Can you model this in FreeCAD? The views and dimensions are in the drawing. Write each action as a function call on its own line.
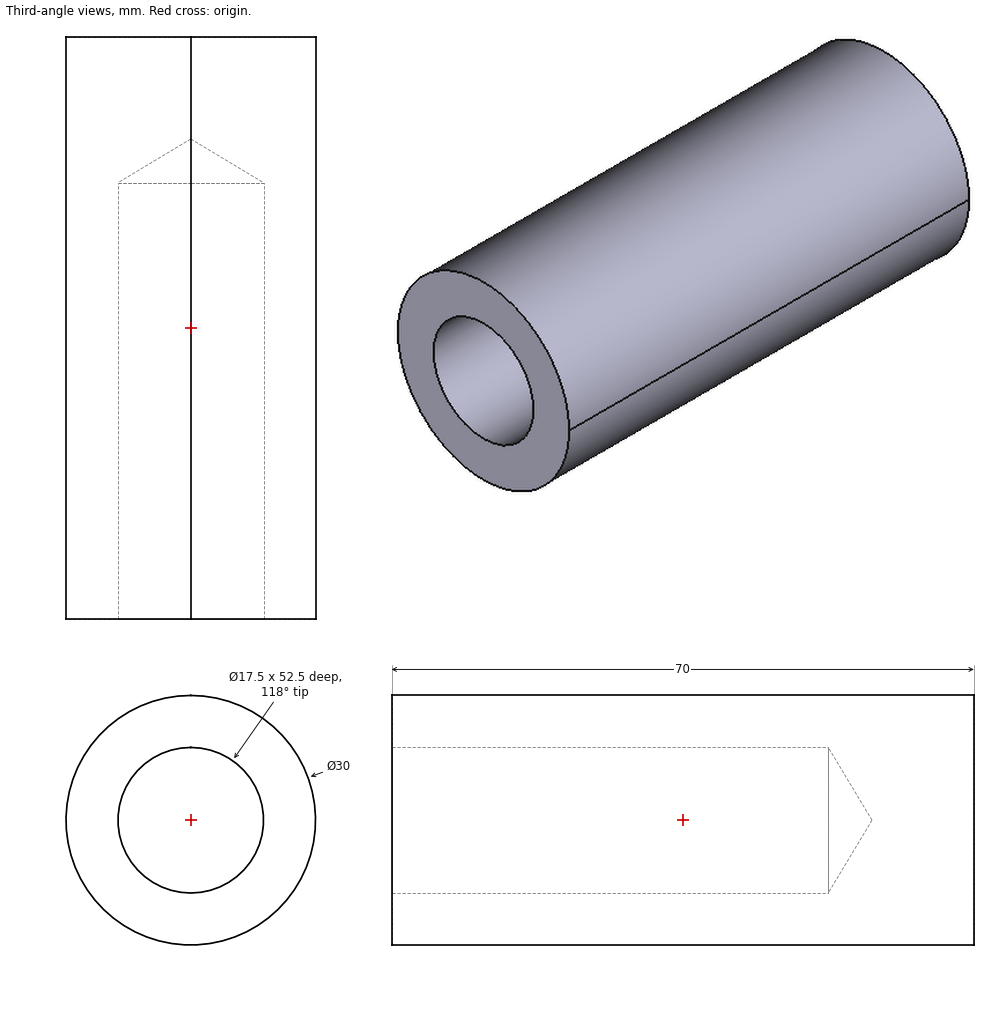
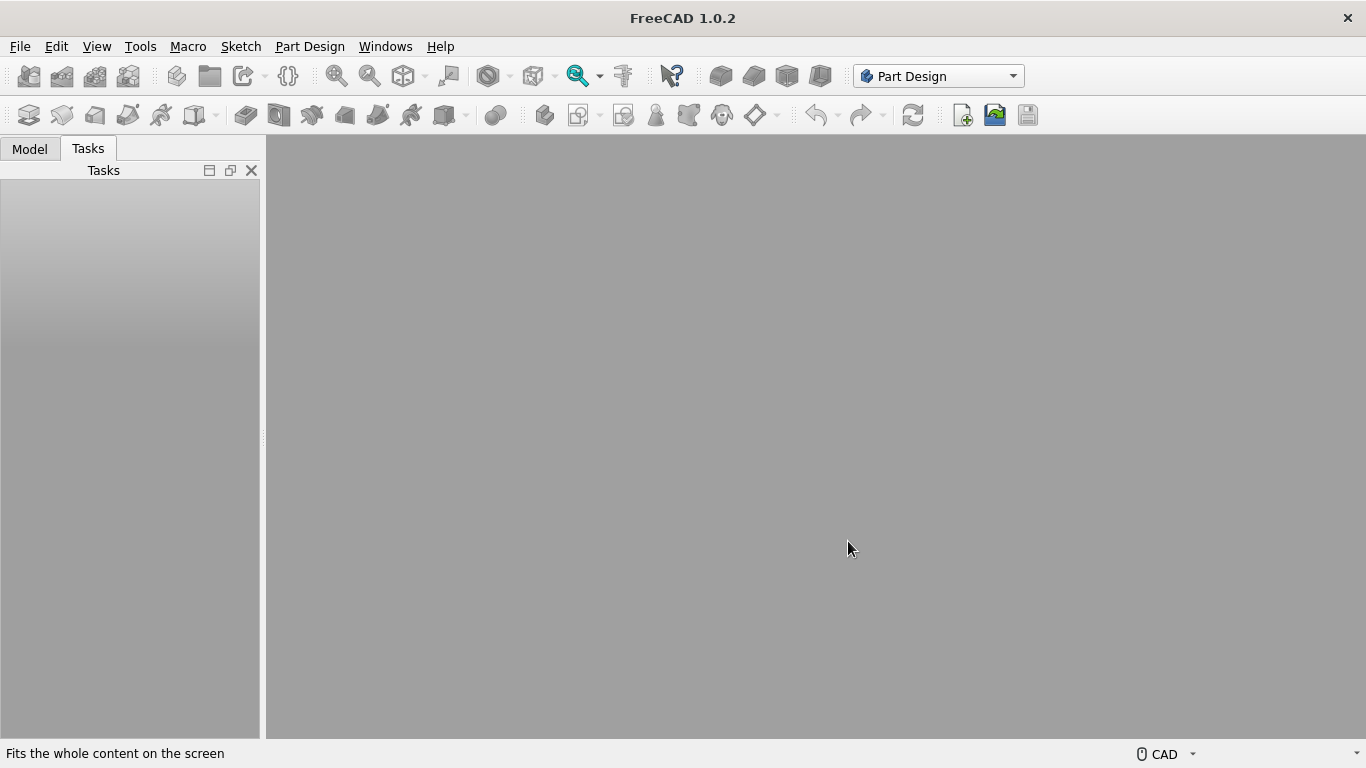
key(ctrl+n)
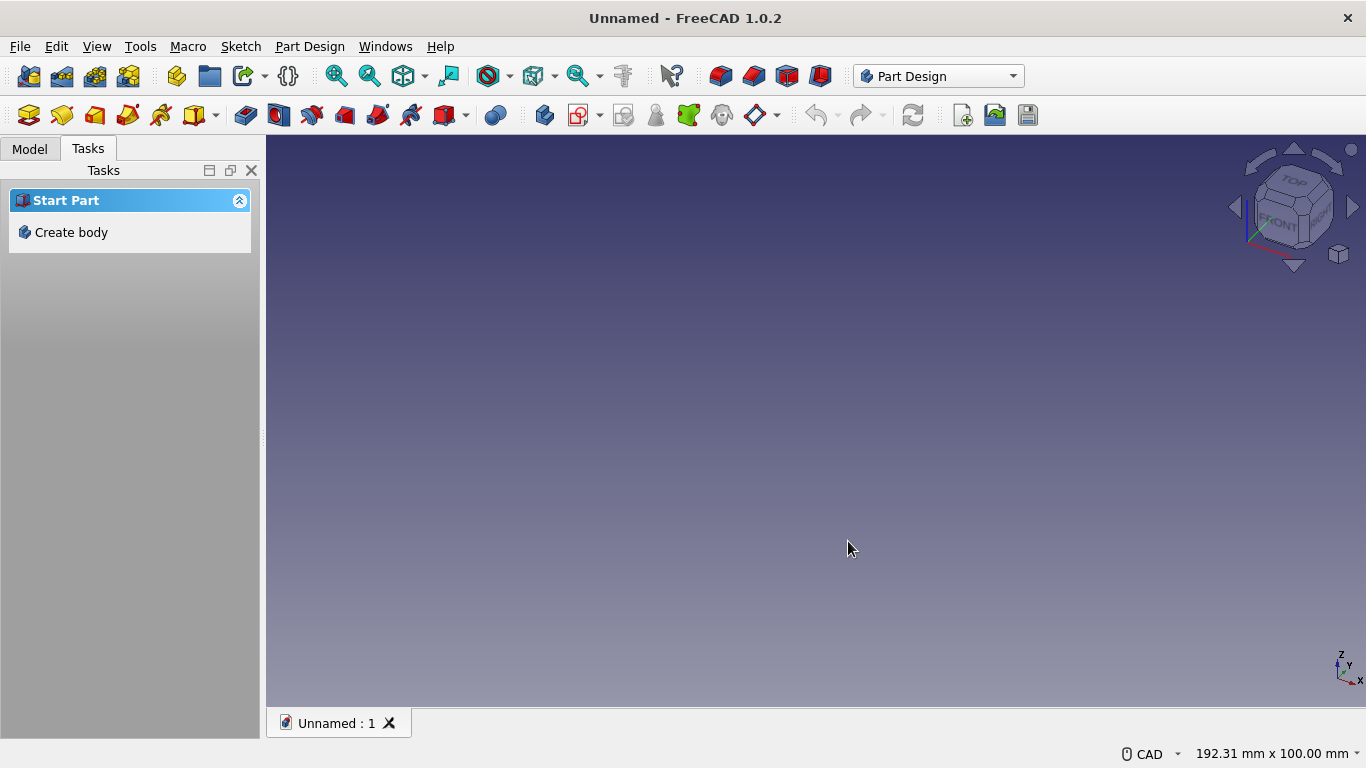
click(578, 116)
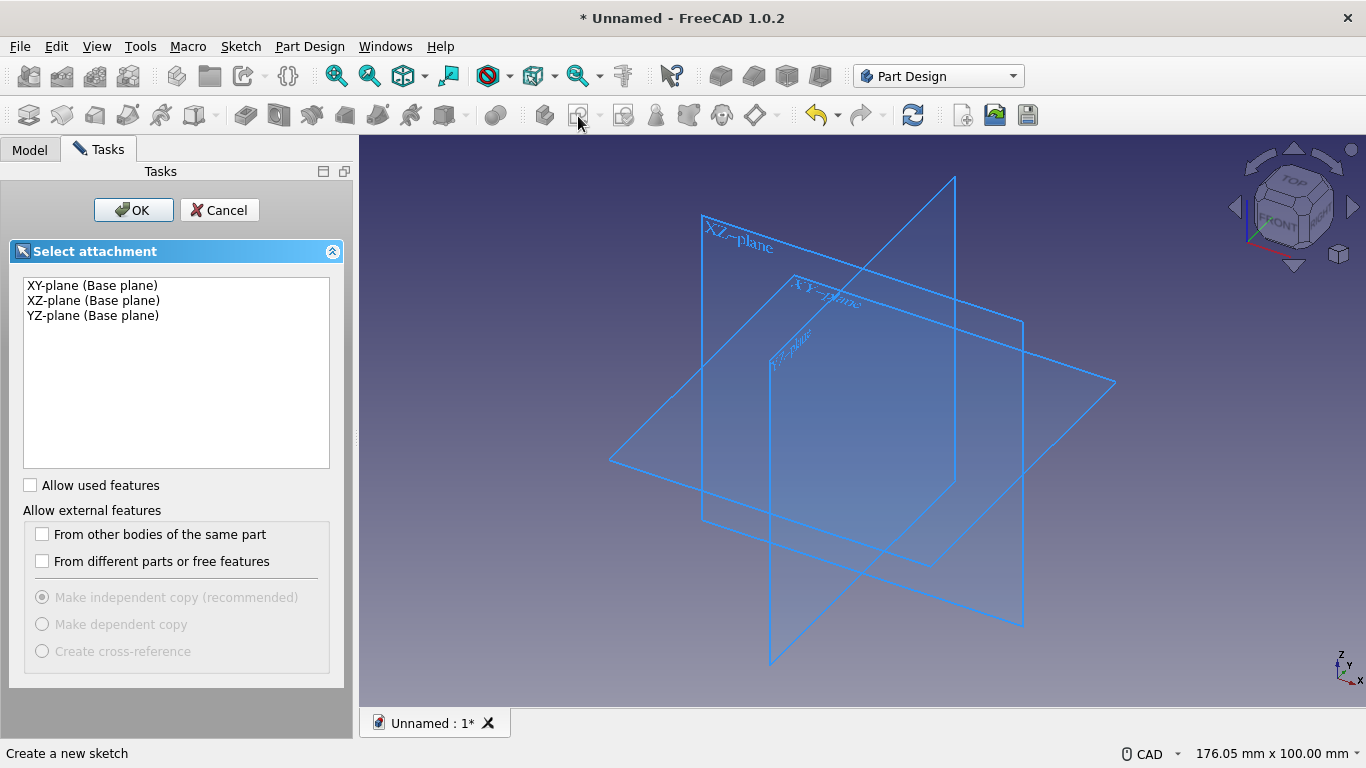
click(84, 300)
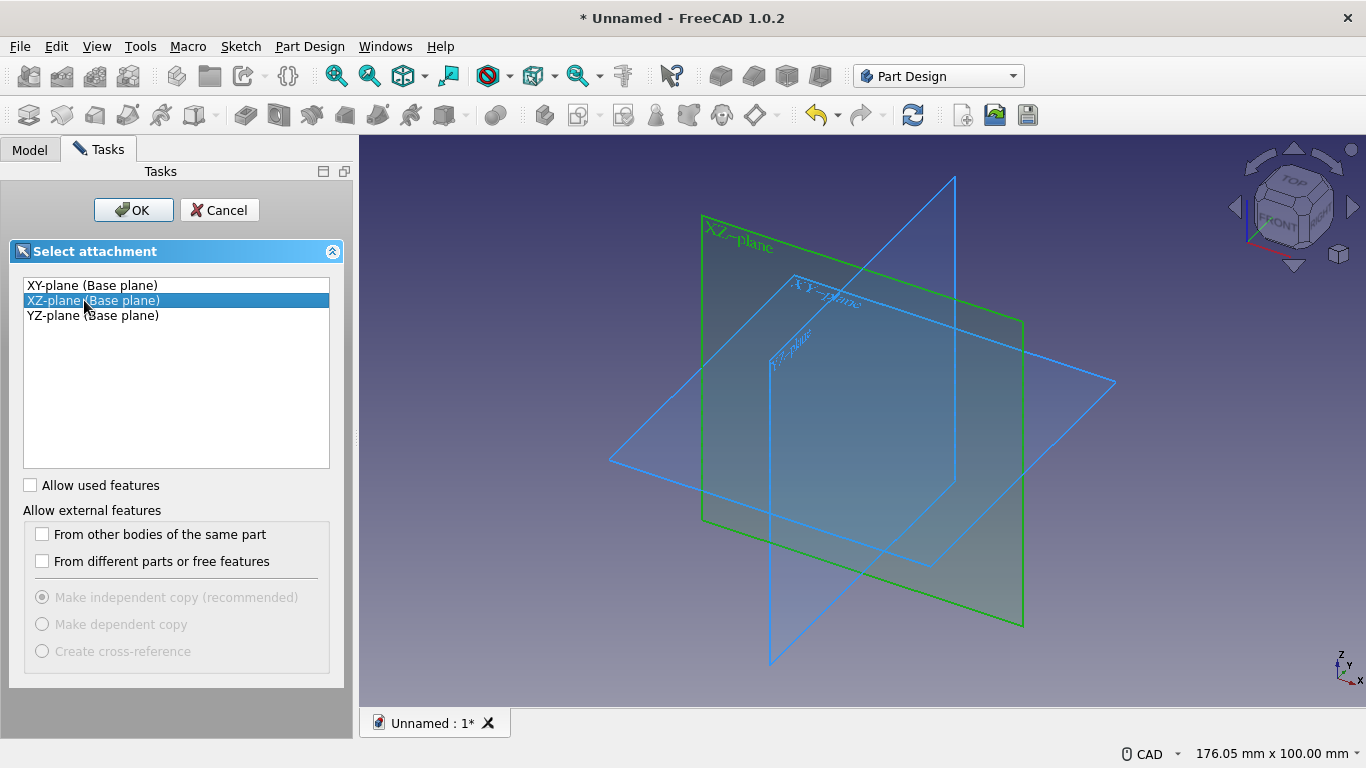
click(134, 210)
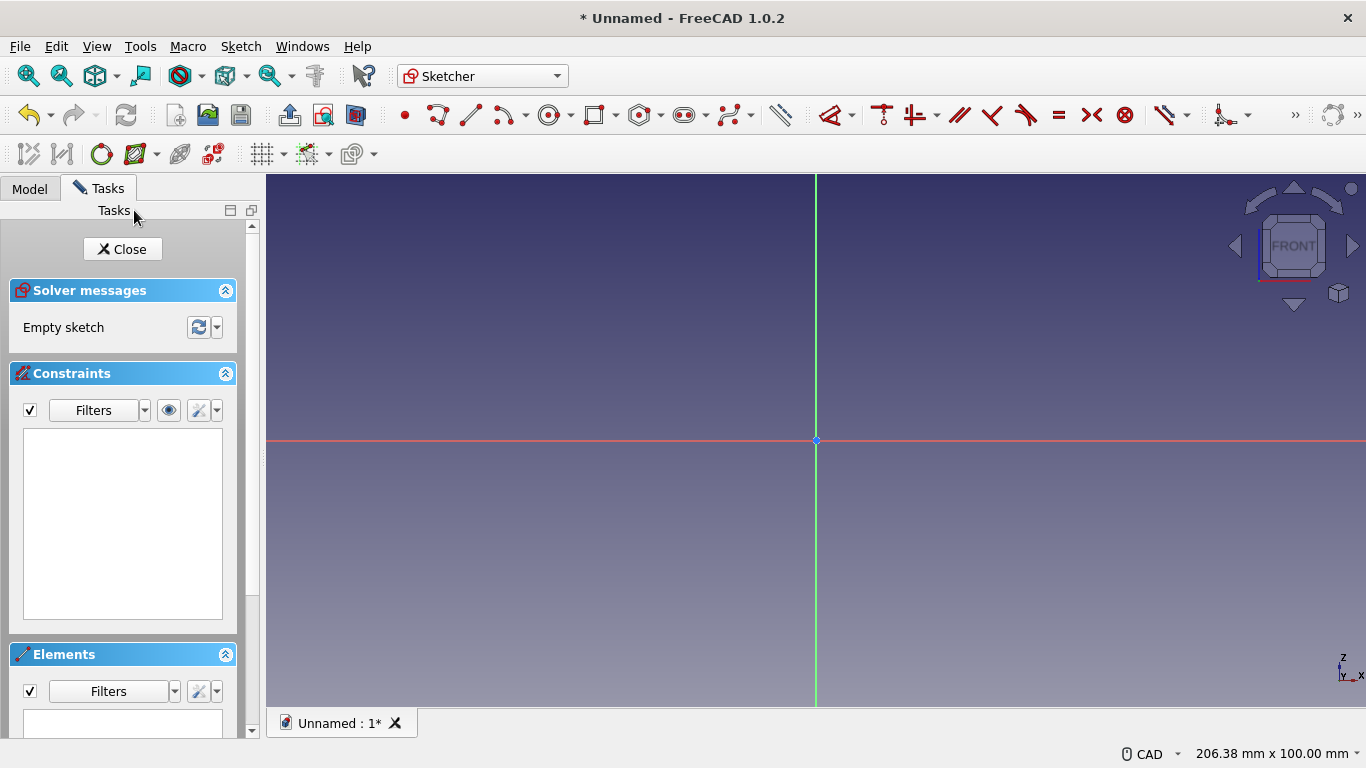
scroll(872, 440, up, 4)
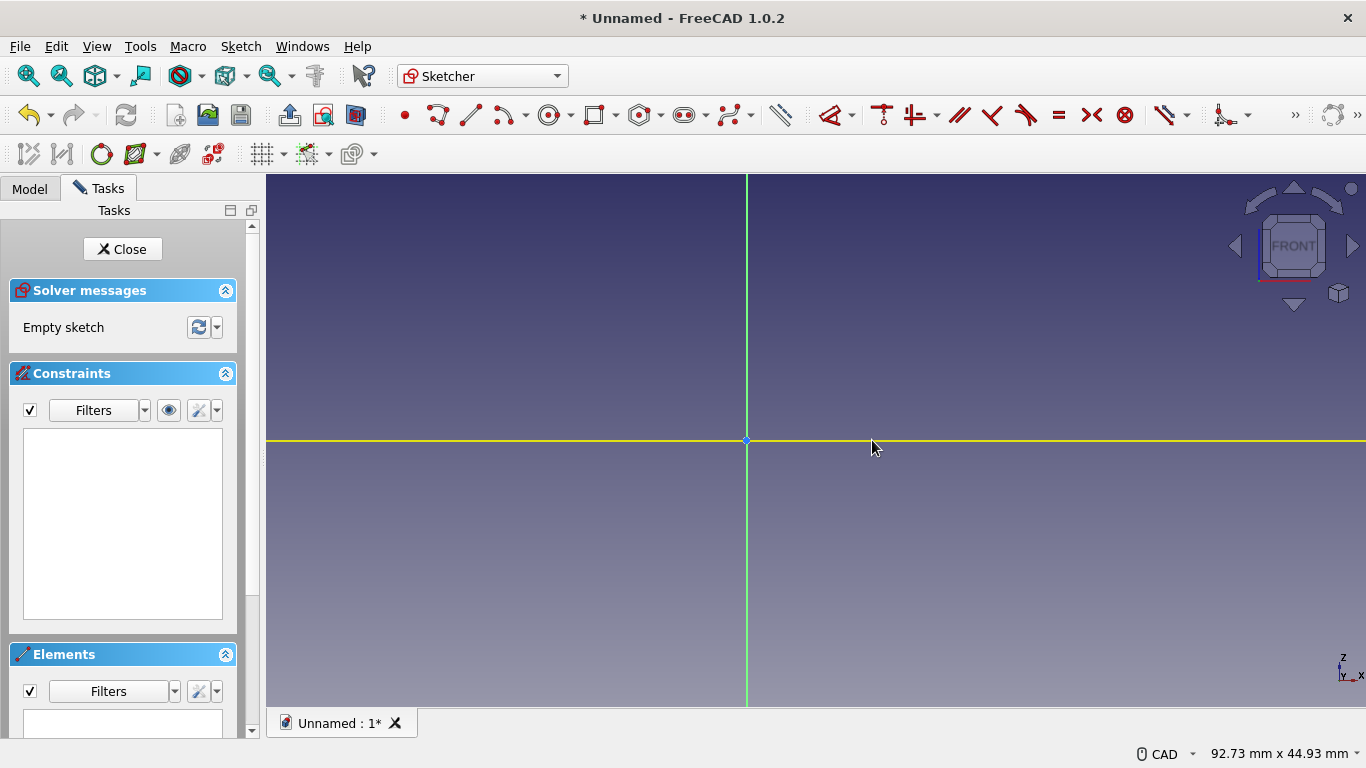
click(548, 116)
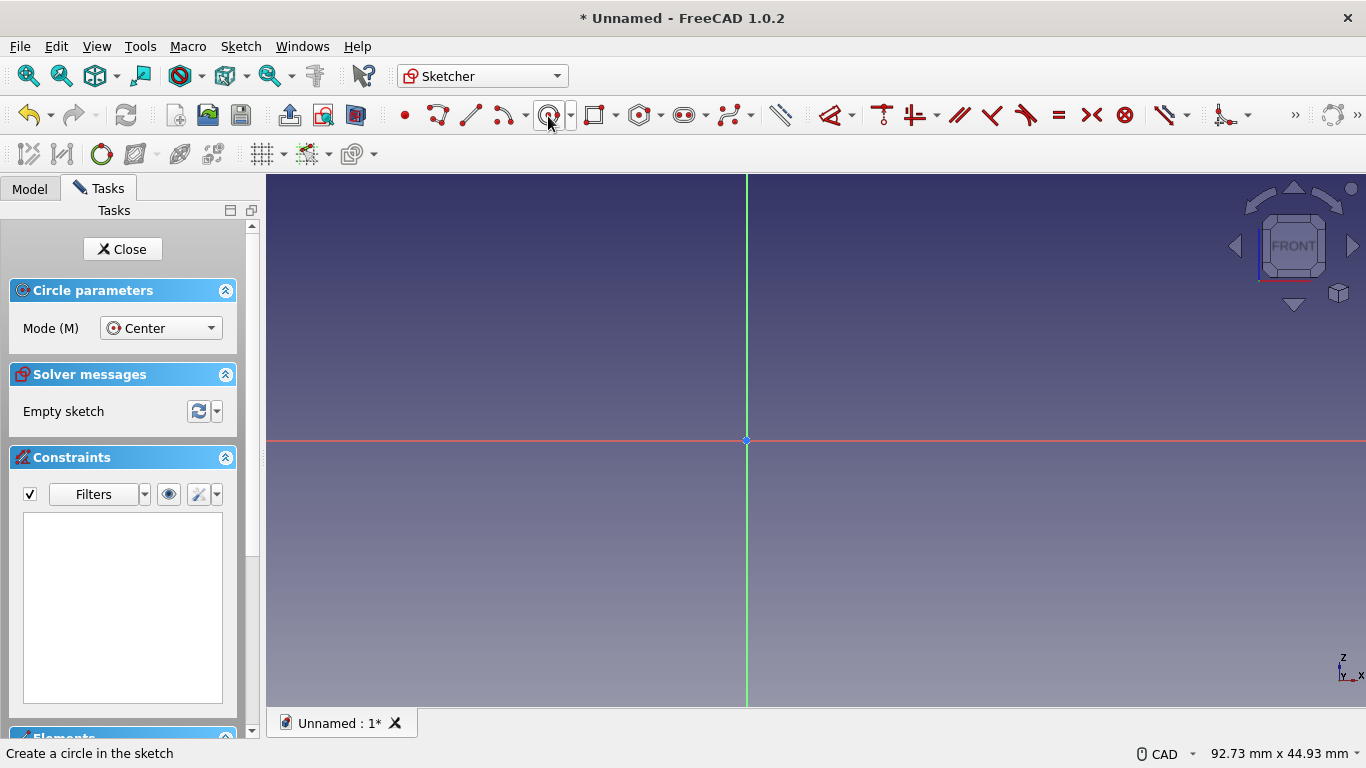
click(747, 440)
click(873, 315)
key(Escape)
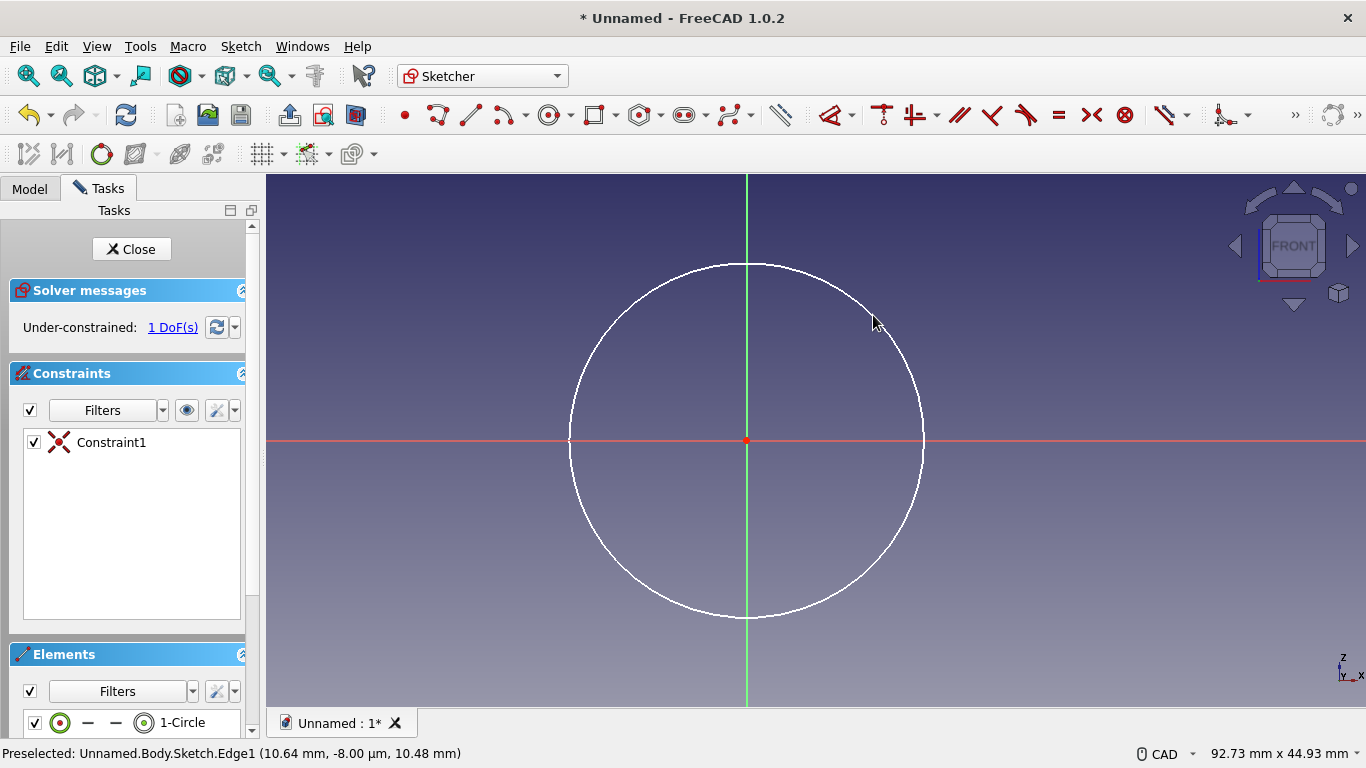
key(d)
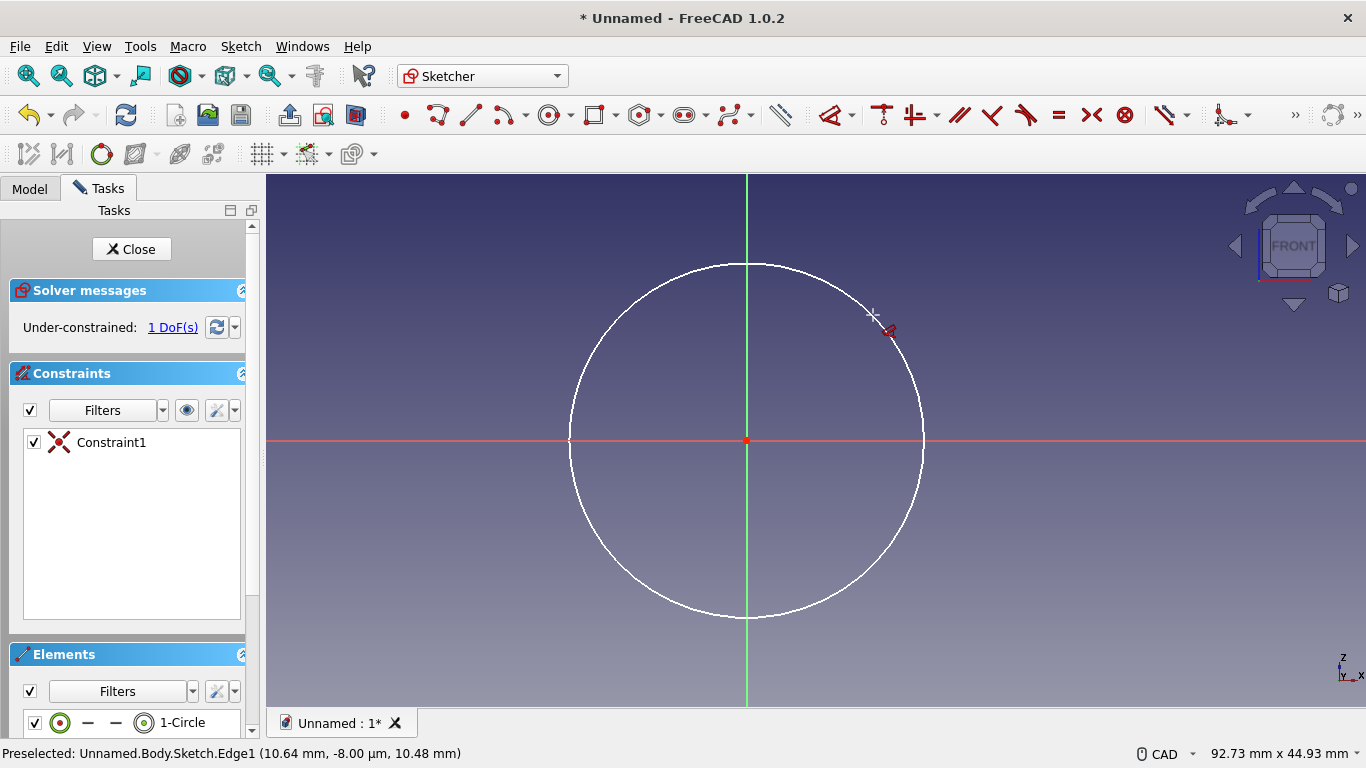
click(872, 315)
click(895, 292)